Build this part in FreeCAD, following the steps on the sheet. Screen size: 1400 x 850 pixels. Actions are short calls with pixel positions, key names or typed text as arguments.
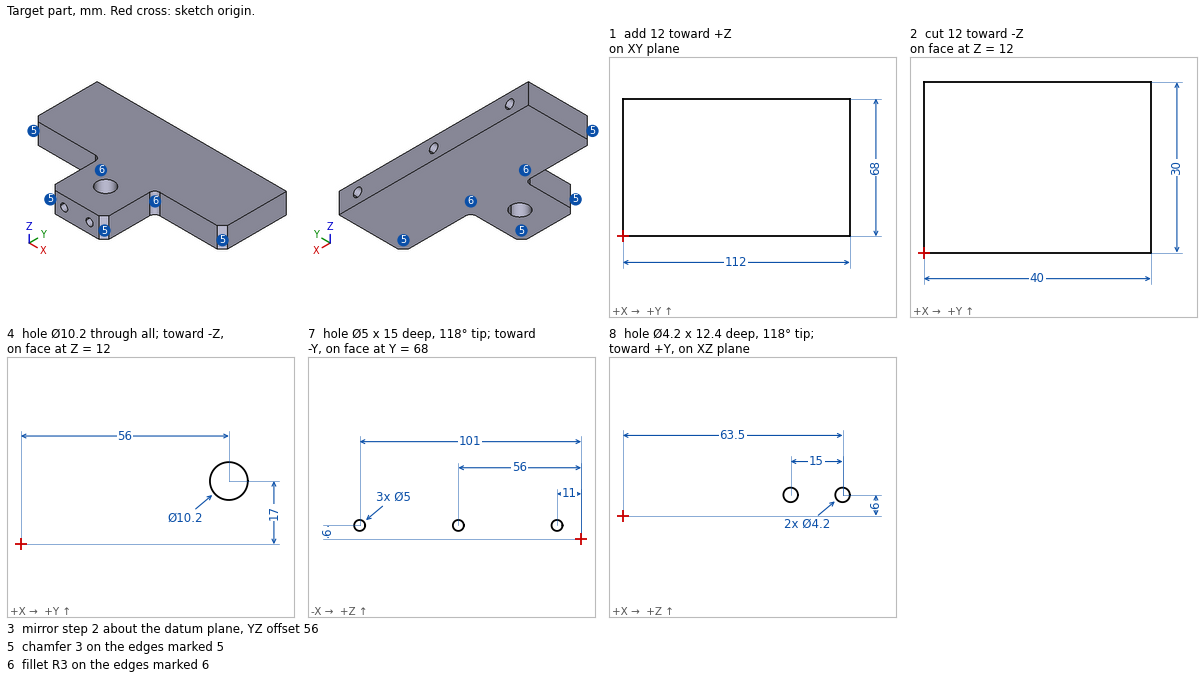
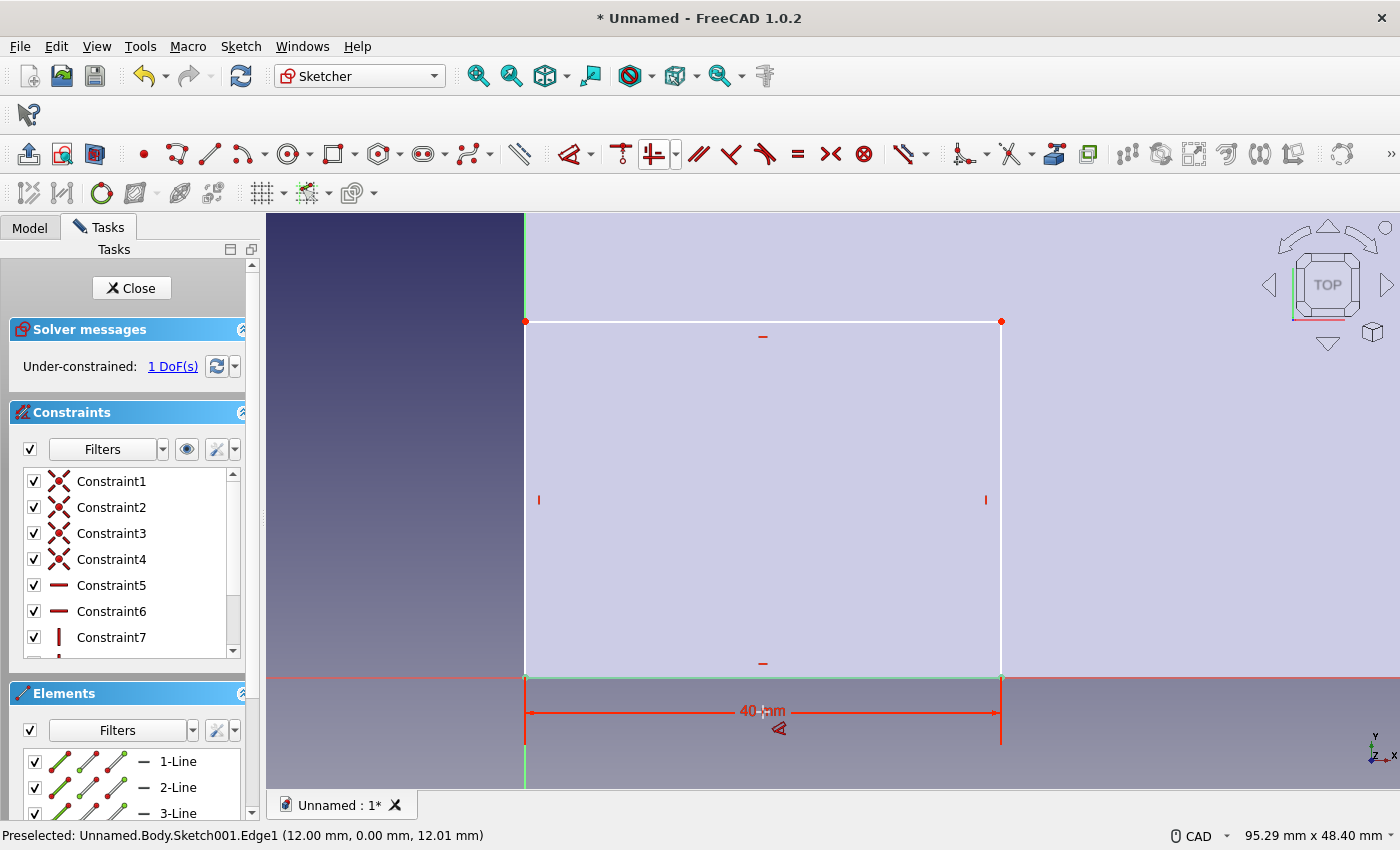
click(1001, 571)
click(1035, 500)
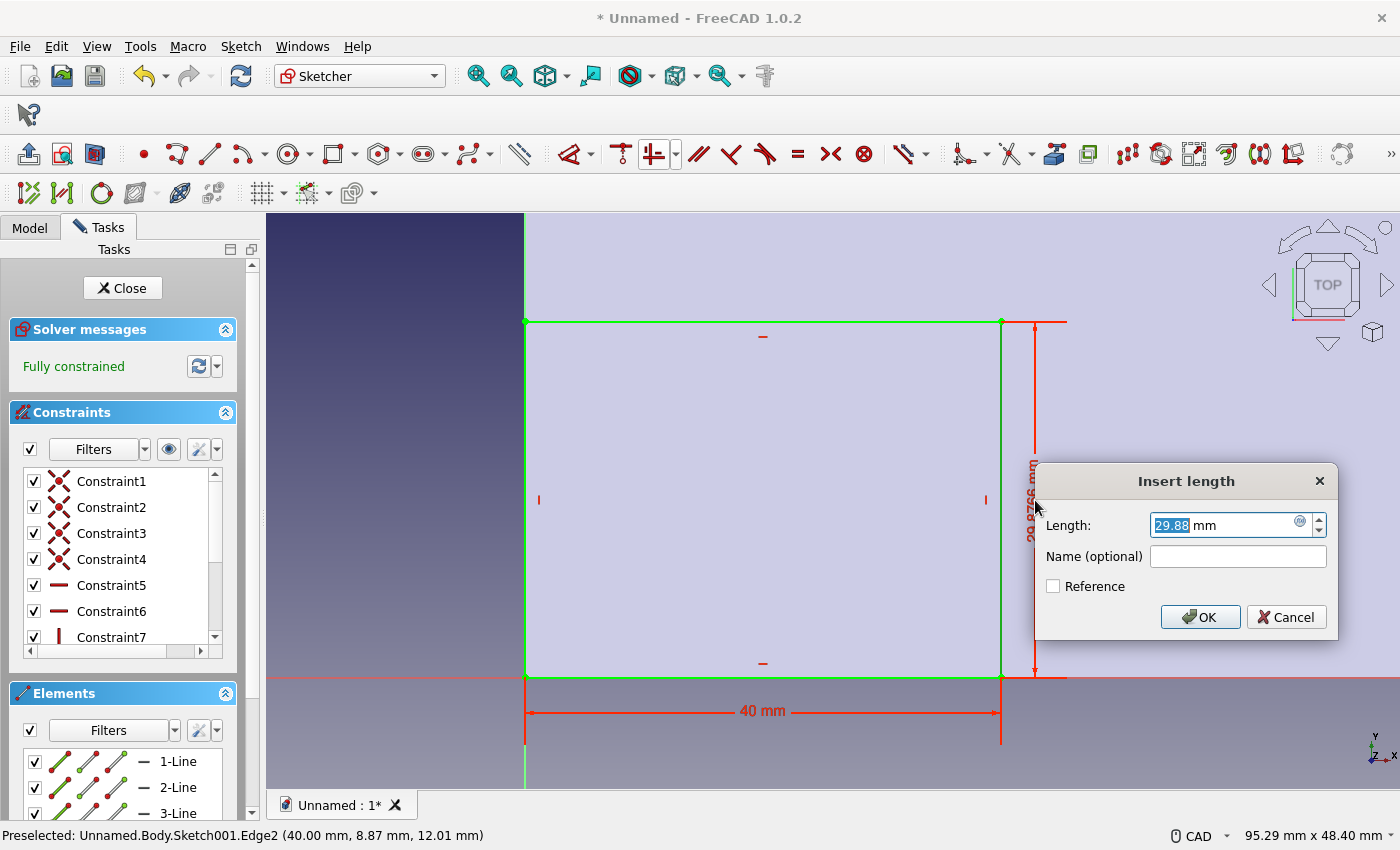
text(30)
key(Return)
key(Escape)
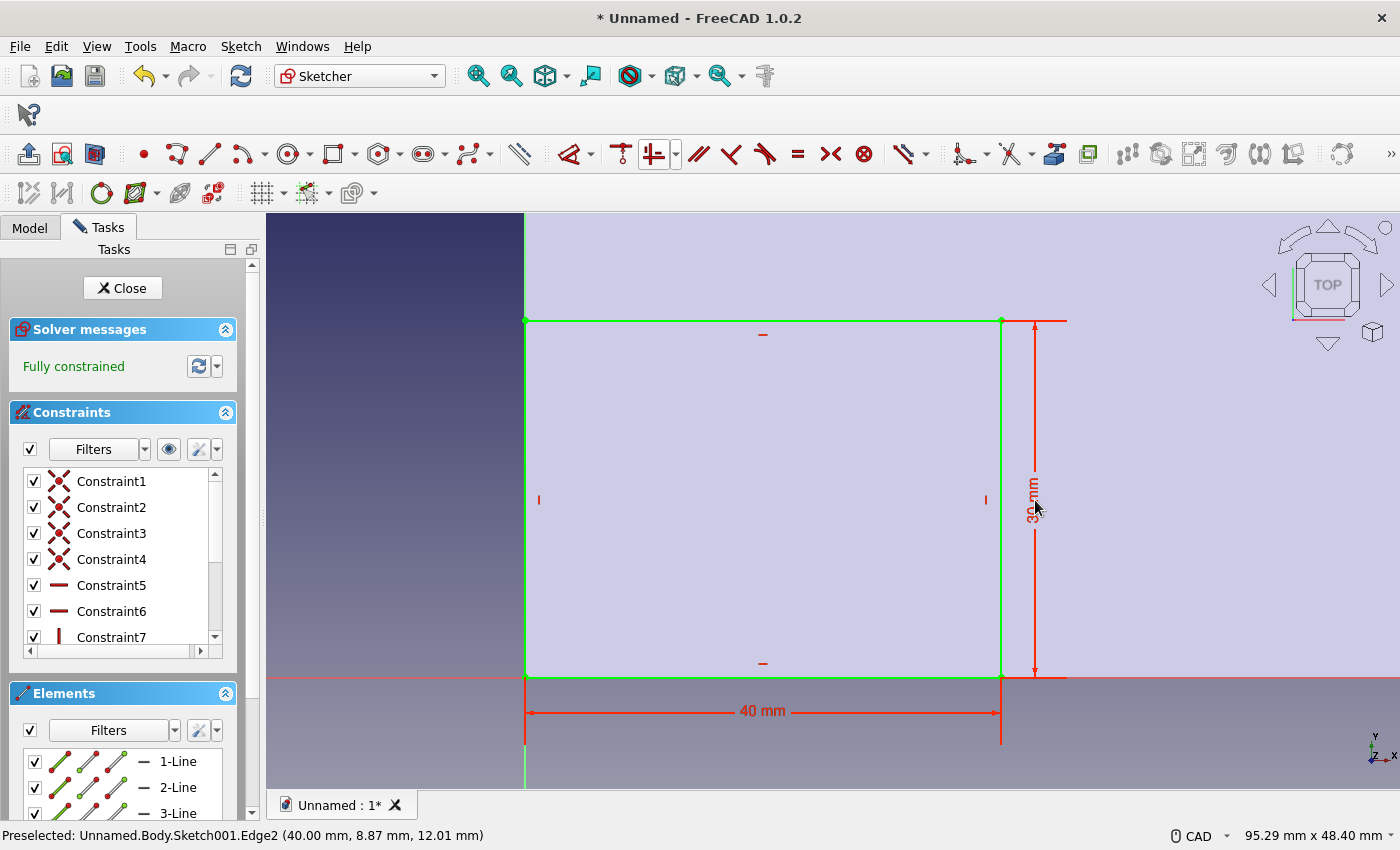
click(123, 288)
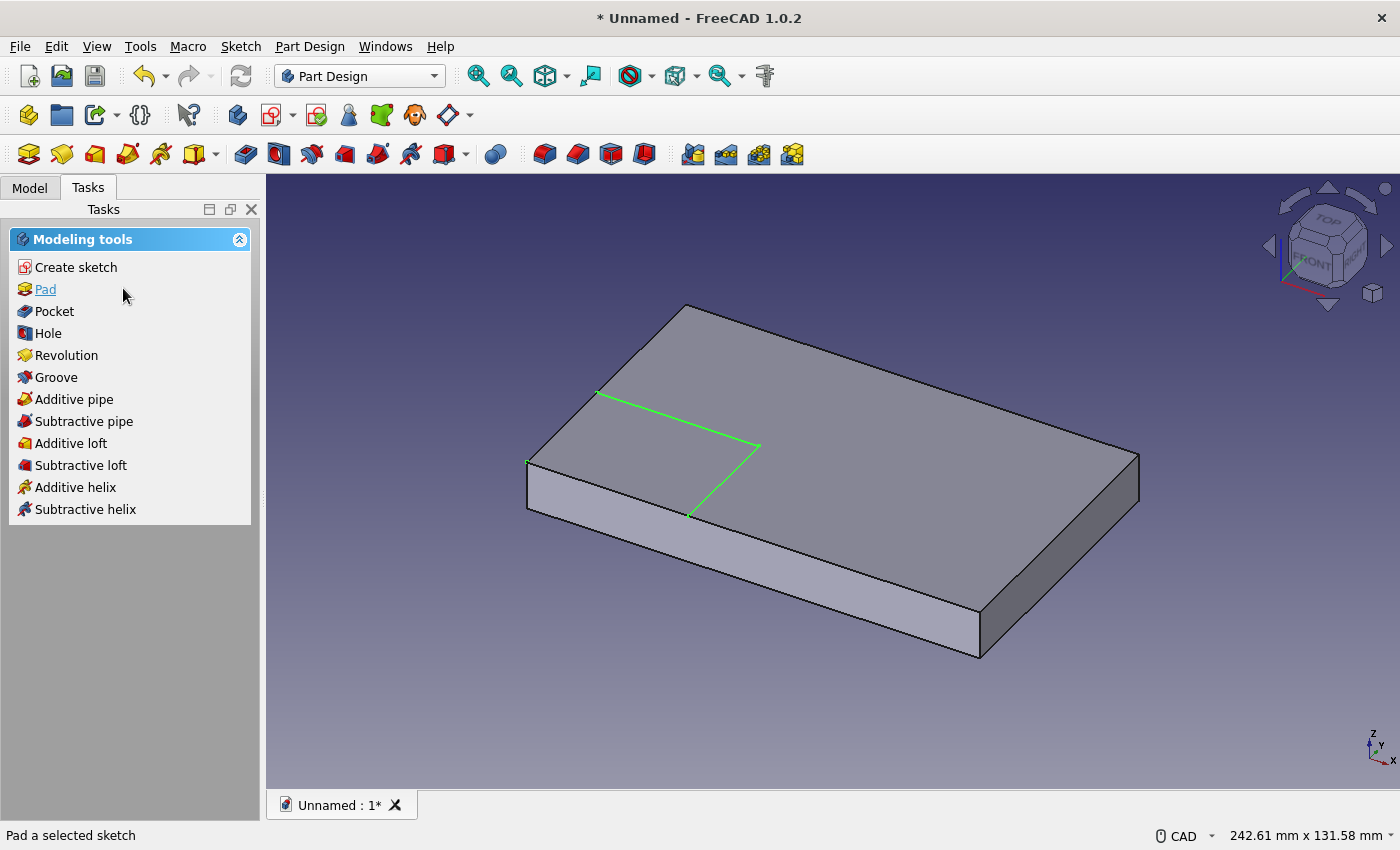
click(246, 154)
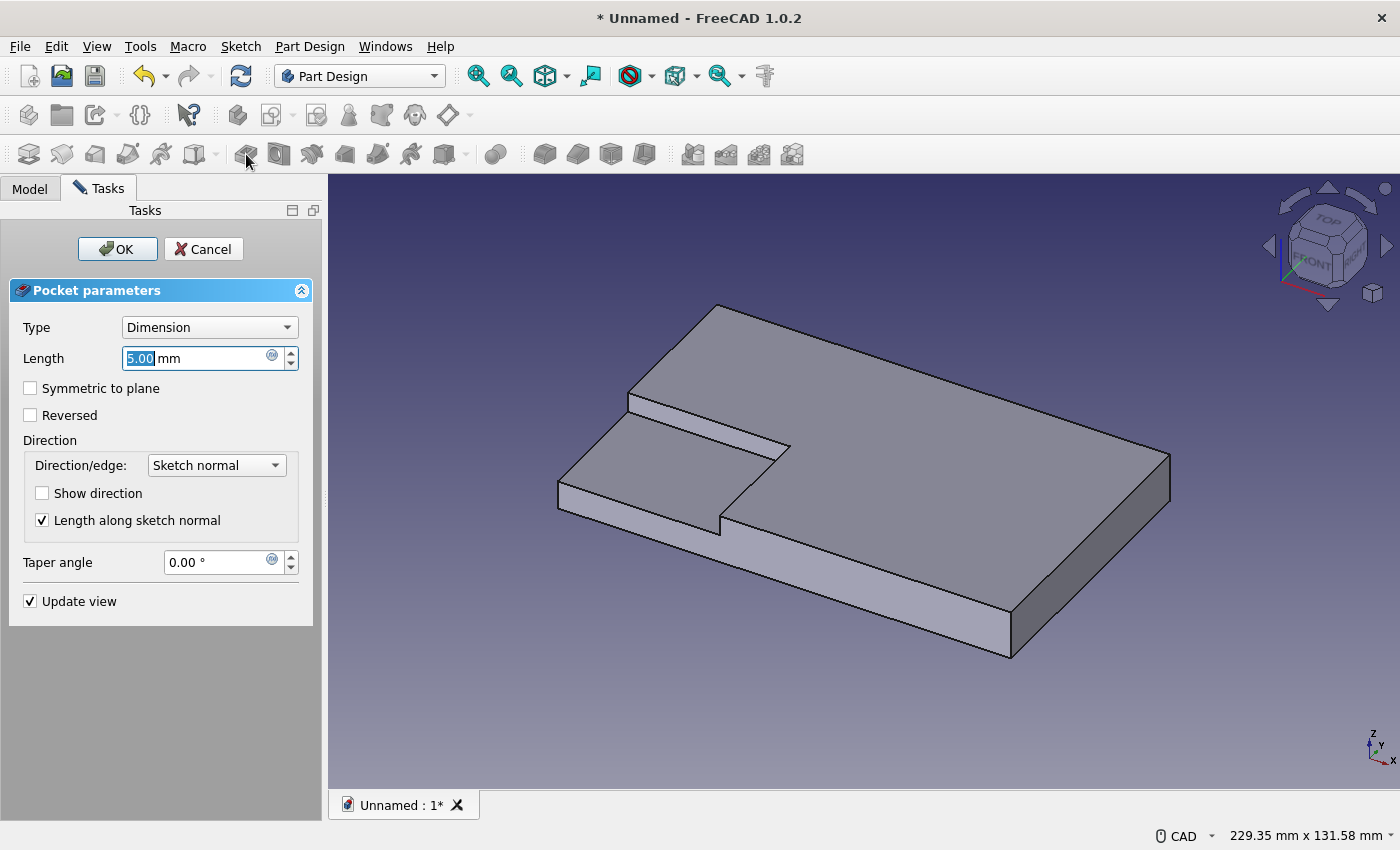
text(12)
key(Tab)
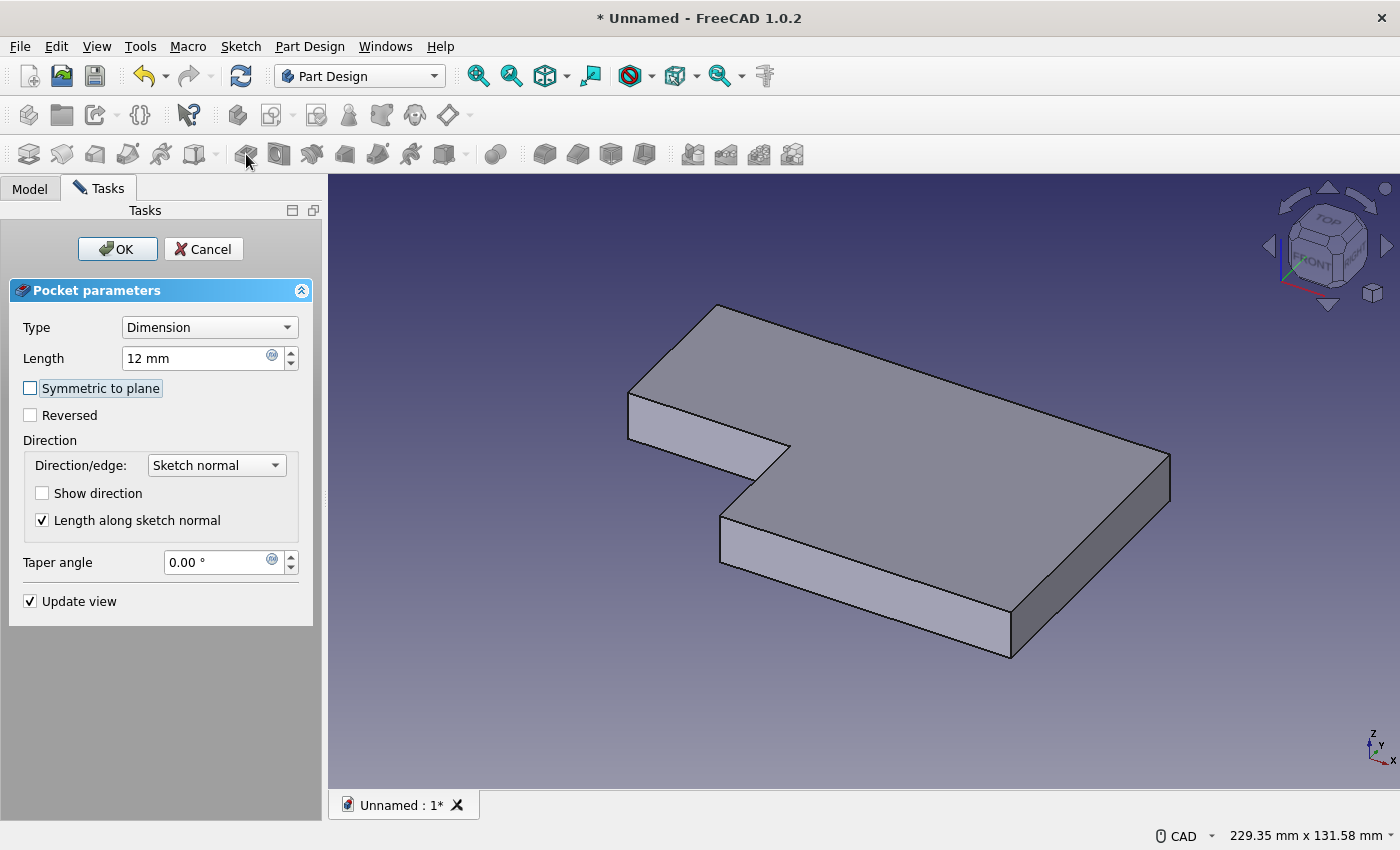
click(118, 249)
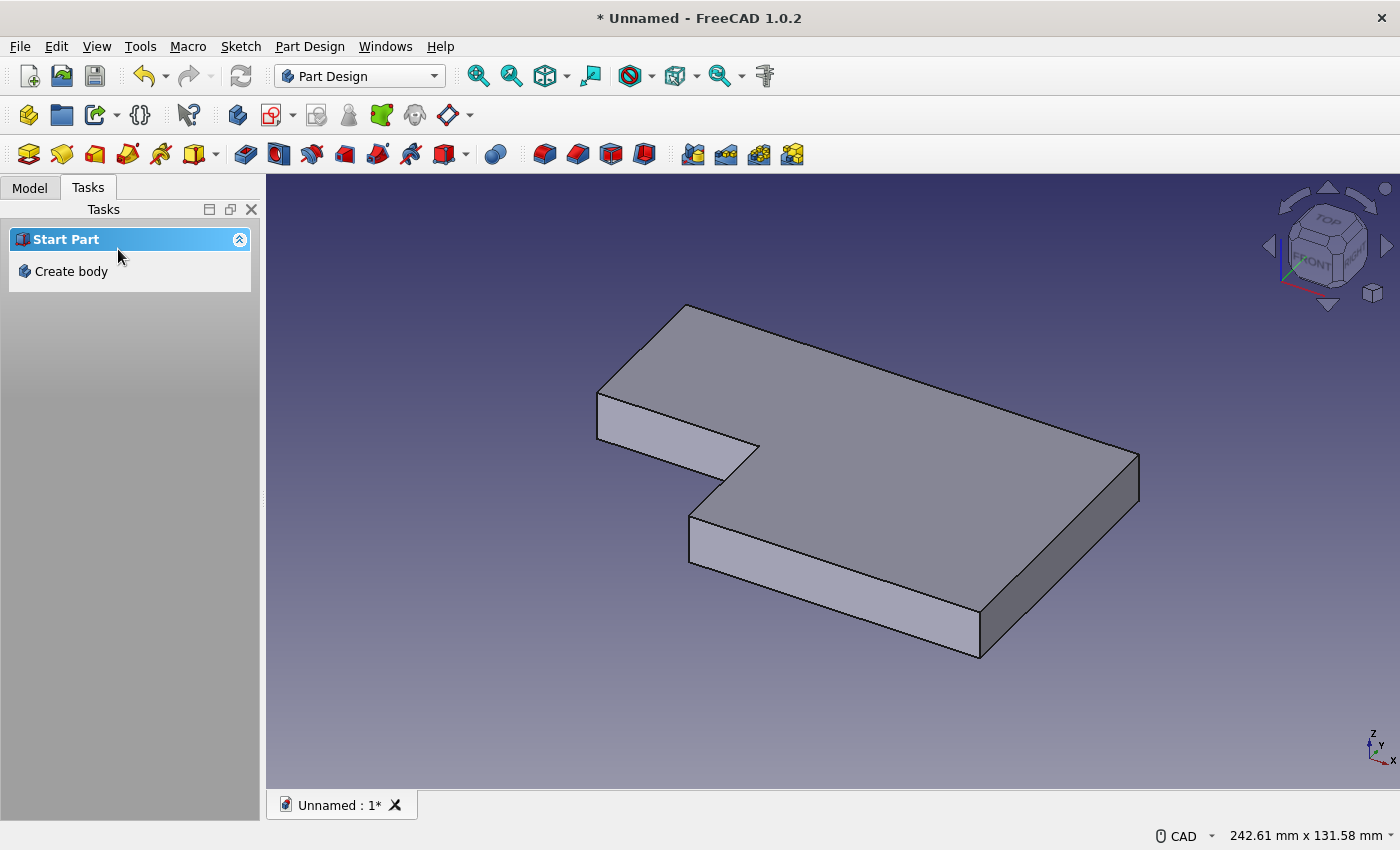
click(30, 188)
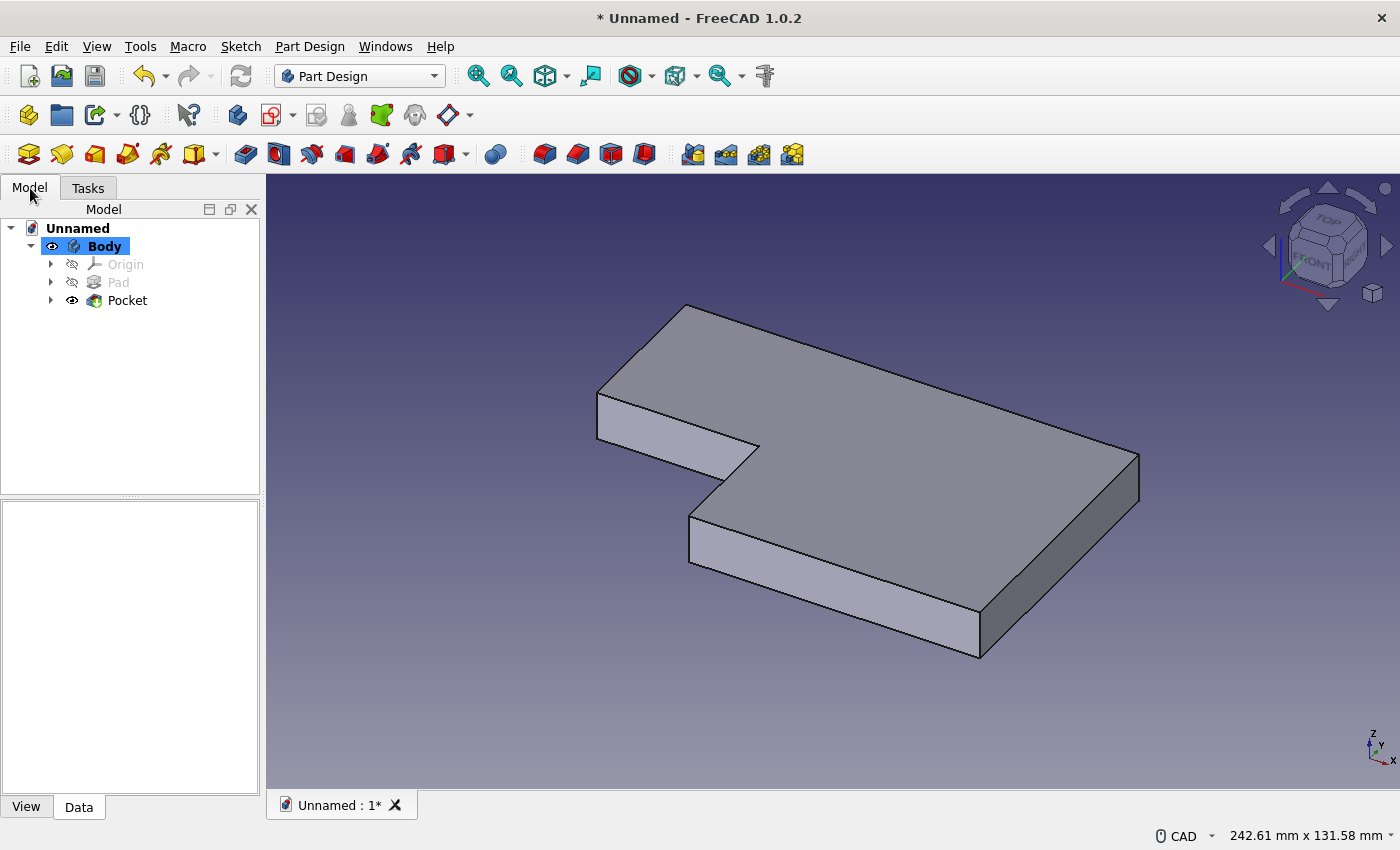
click(51, 264)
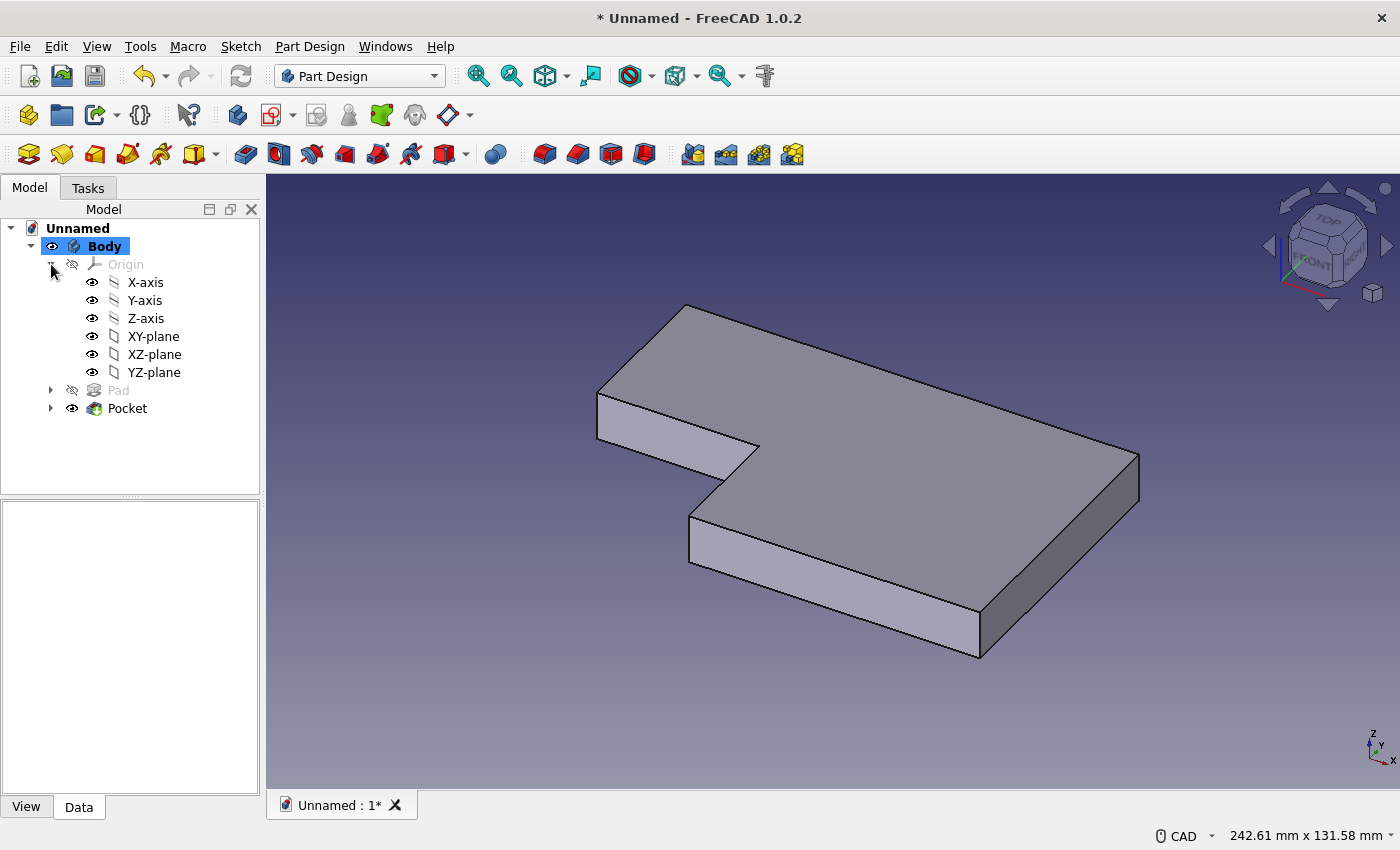
click(137, 372)